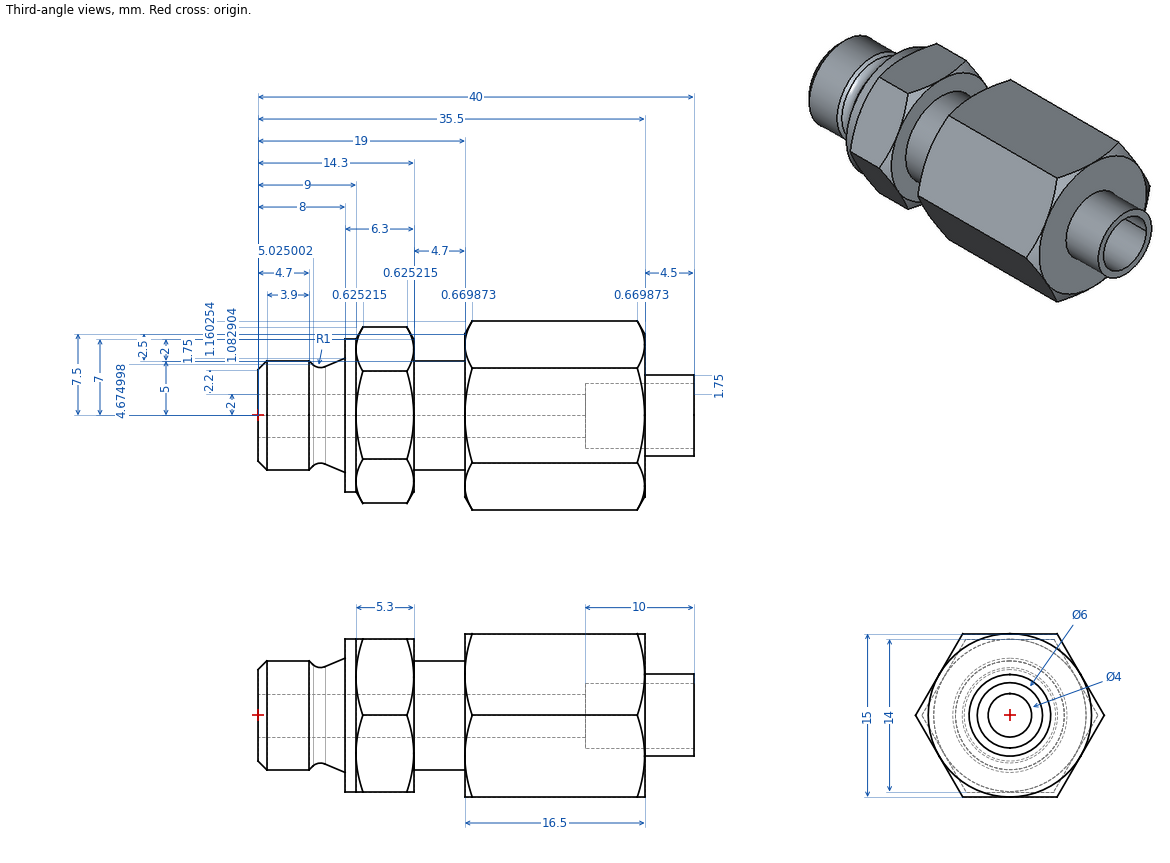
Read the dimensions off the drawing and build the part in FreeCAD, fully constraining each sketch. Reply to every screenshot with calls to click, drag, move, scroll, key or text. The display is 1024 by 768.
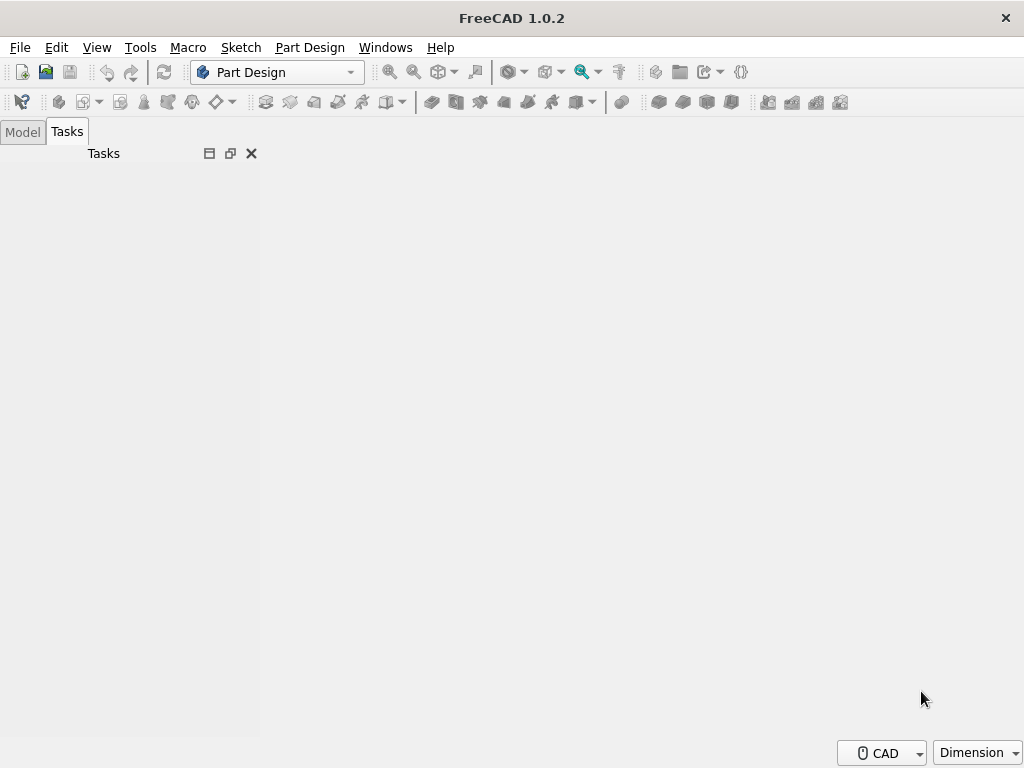
key(ctrl+n)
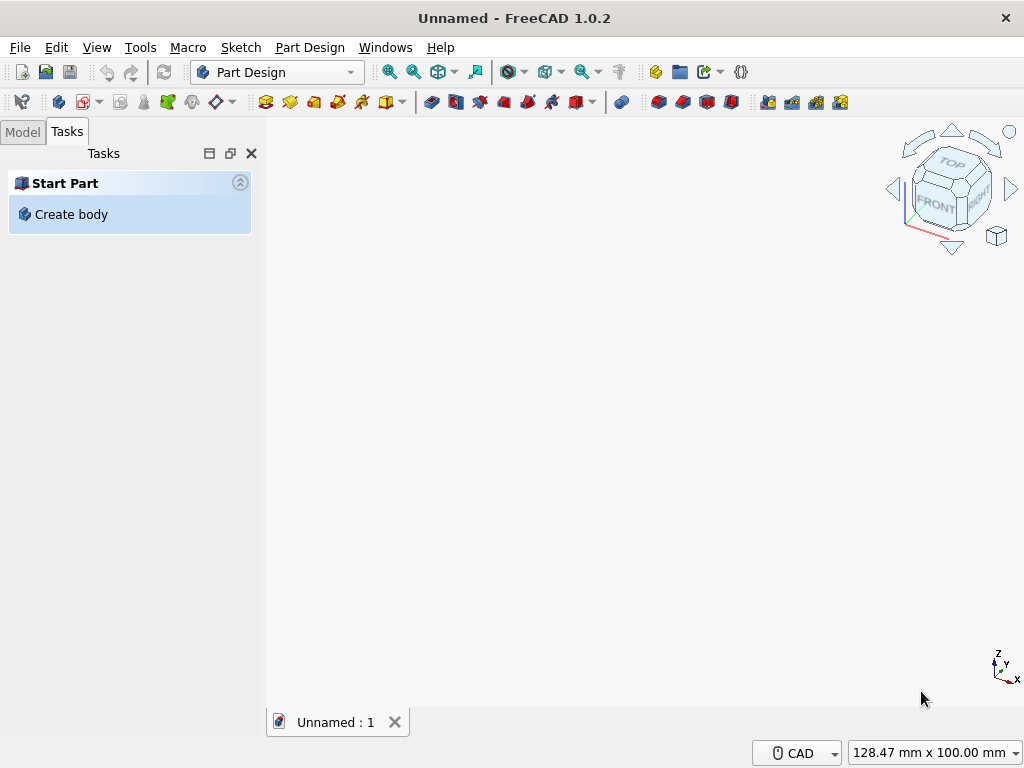
click(84, 102)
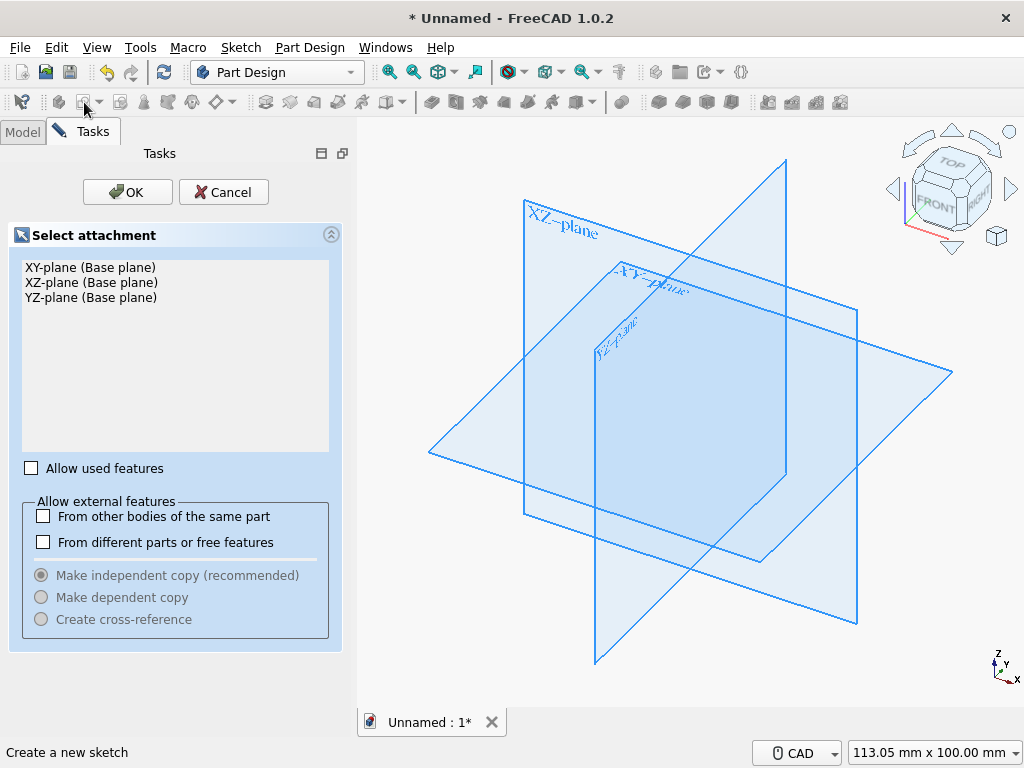
click(82, 268)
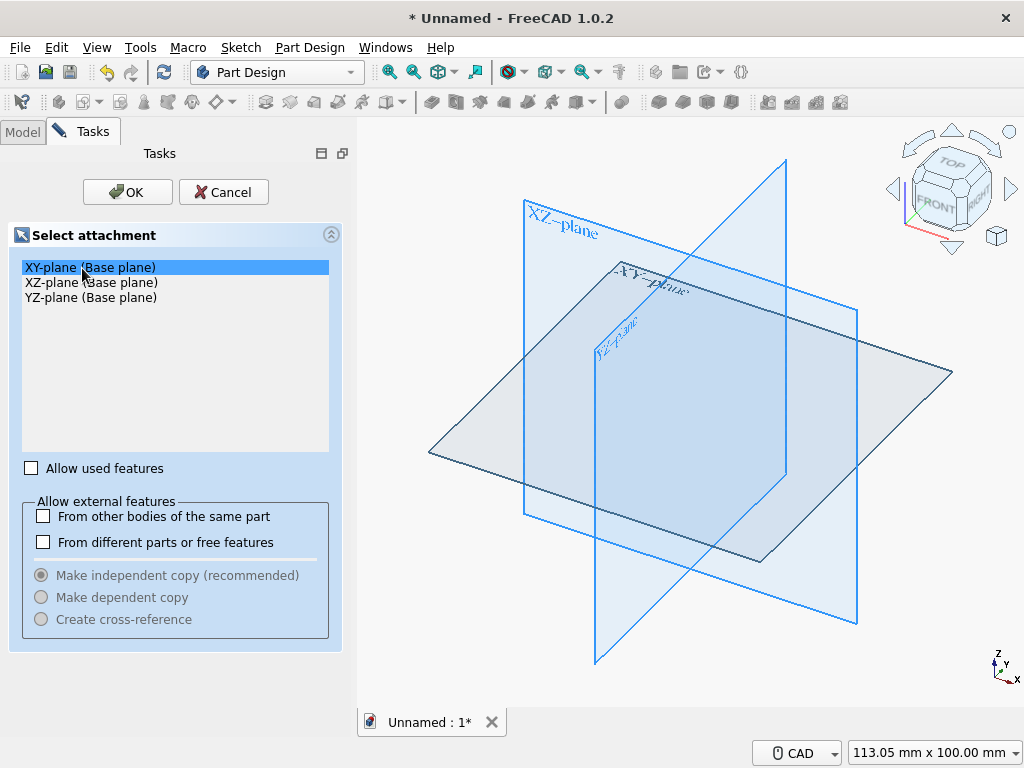
click(128, 192)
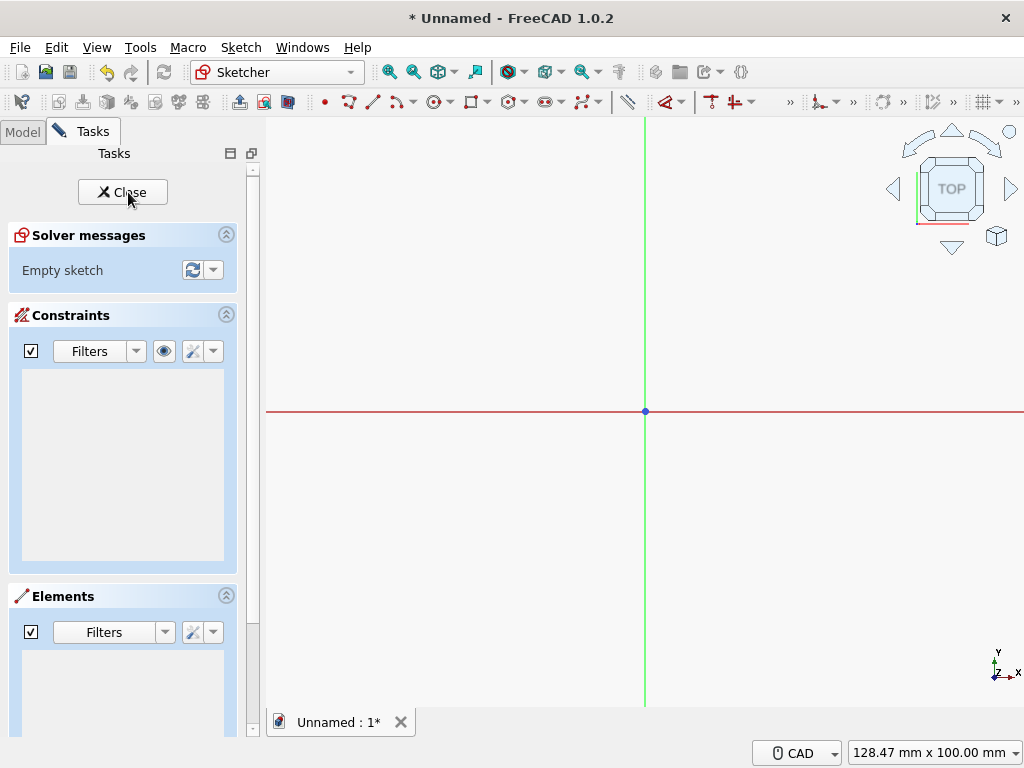
scroll(576, 412, down, 5)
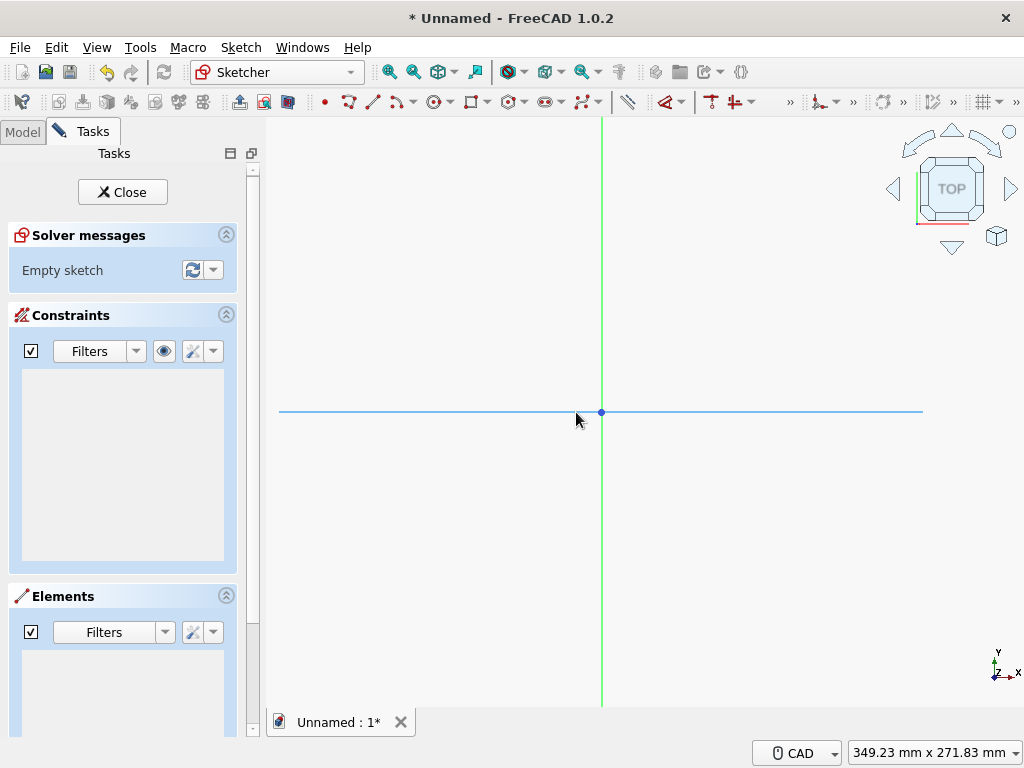
scroll(662, 402, up, 8)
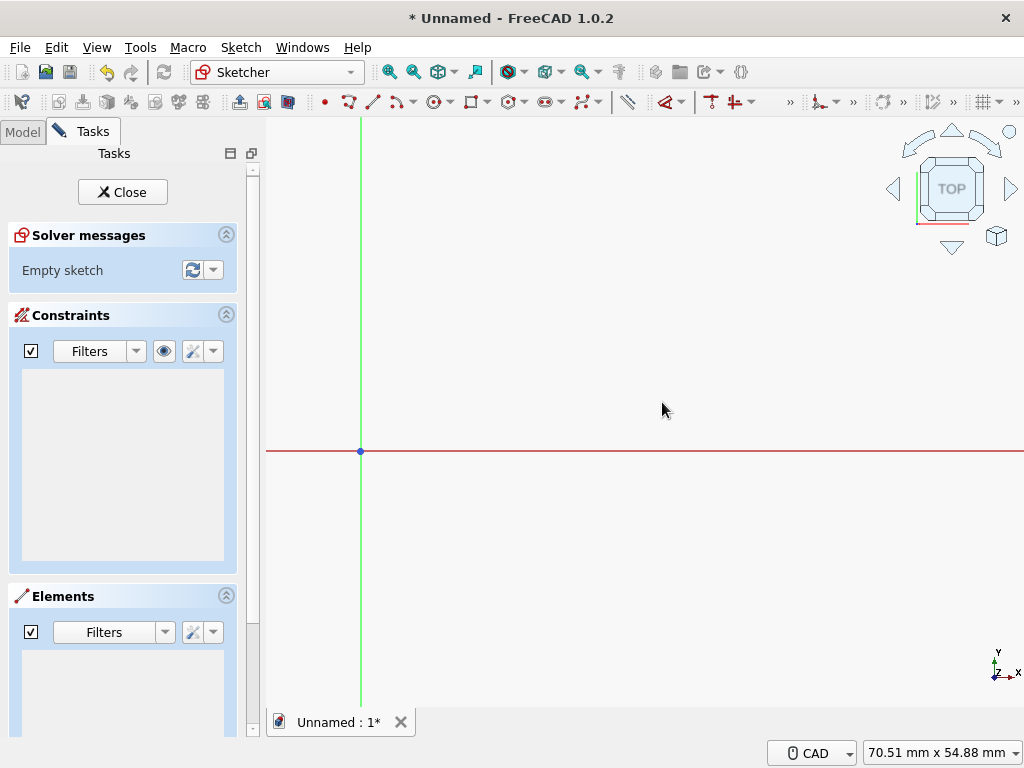
key(g)
key(m)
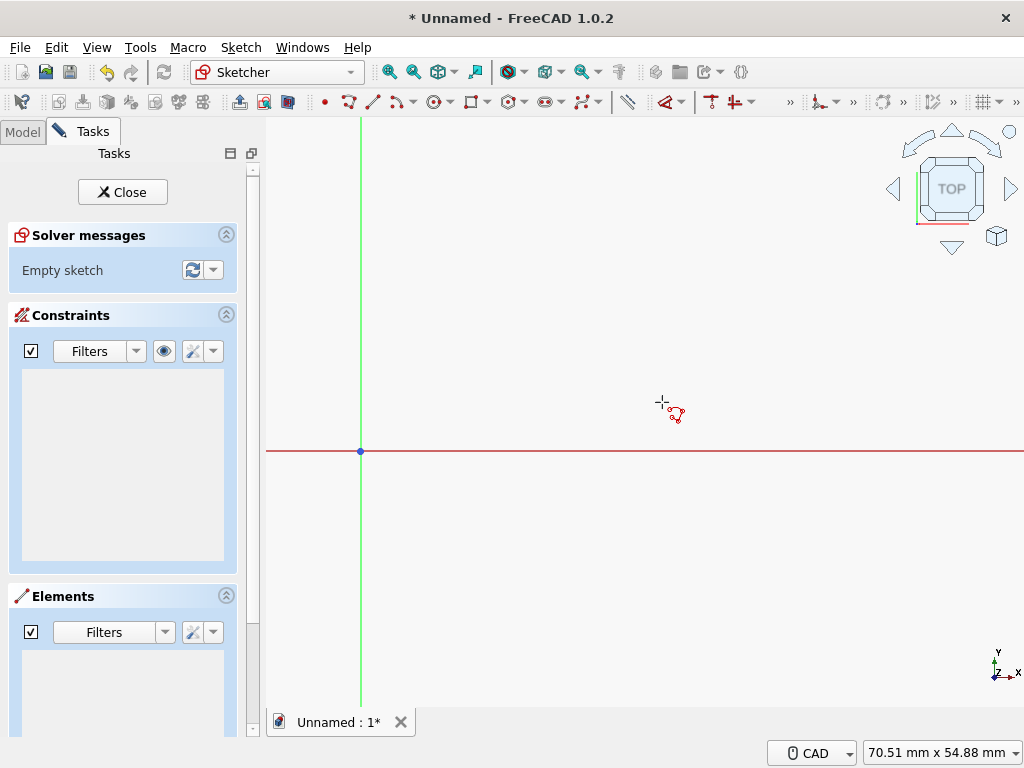
click(415, 401)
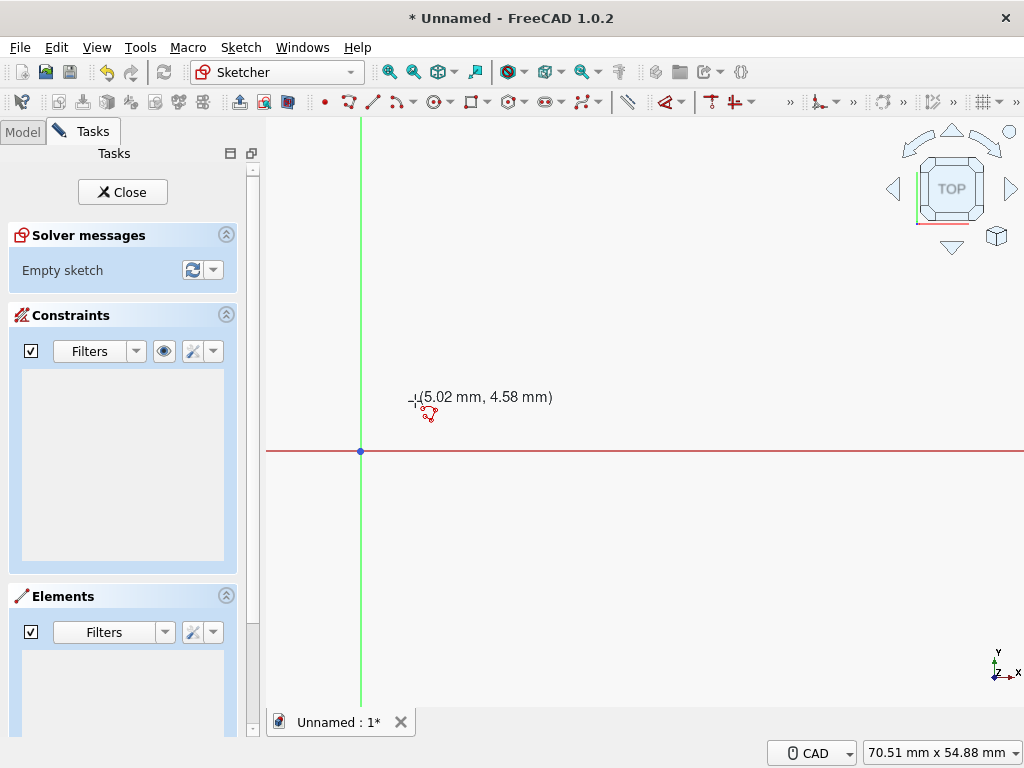
scroll(412, 397, up, 6)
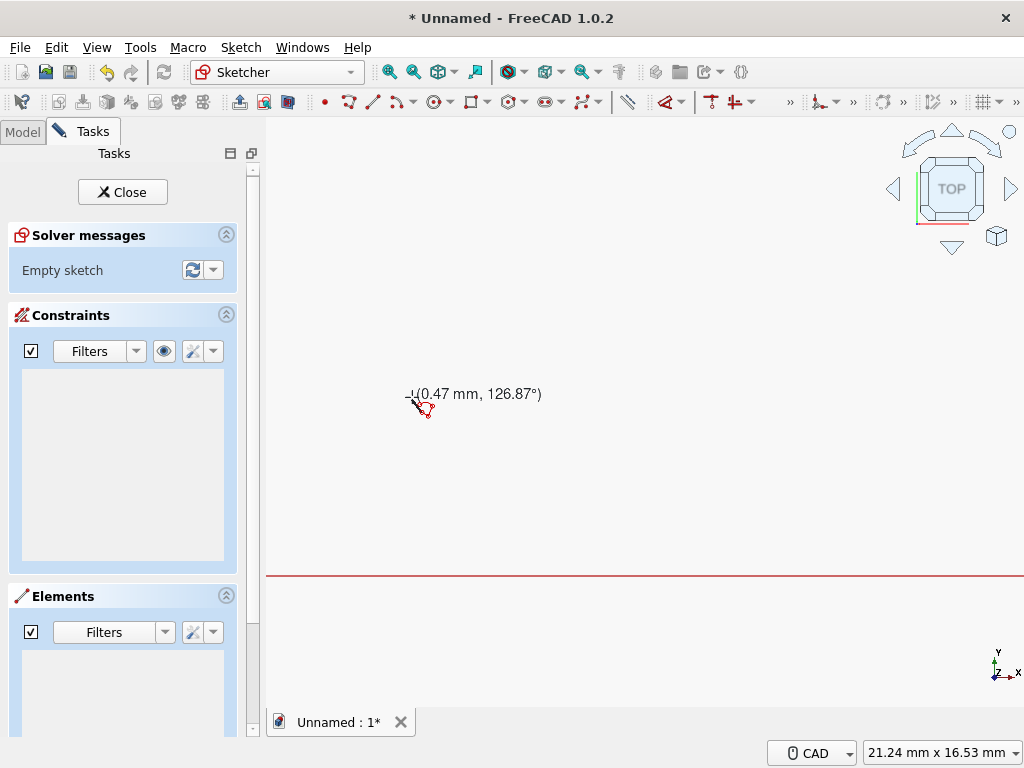
click(410, 397)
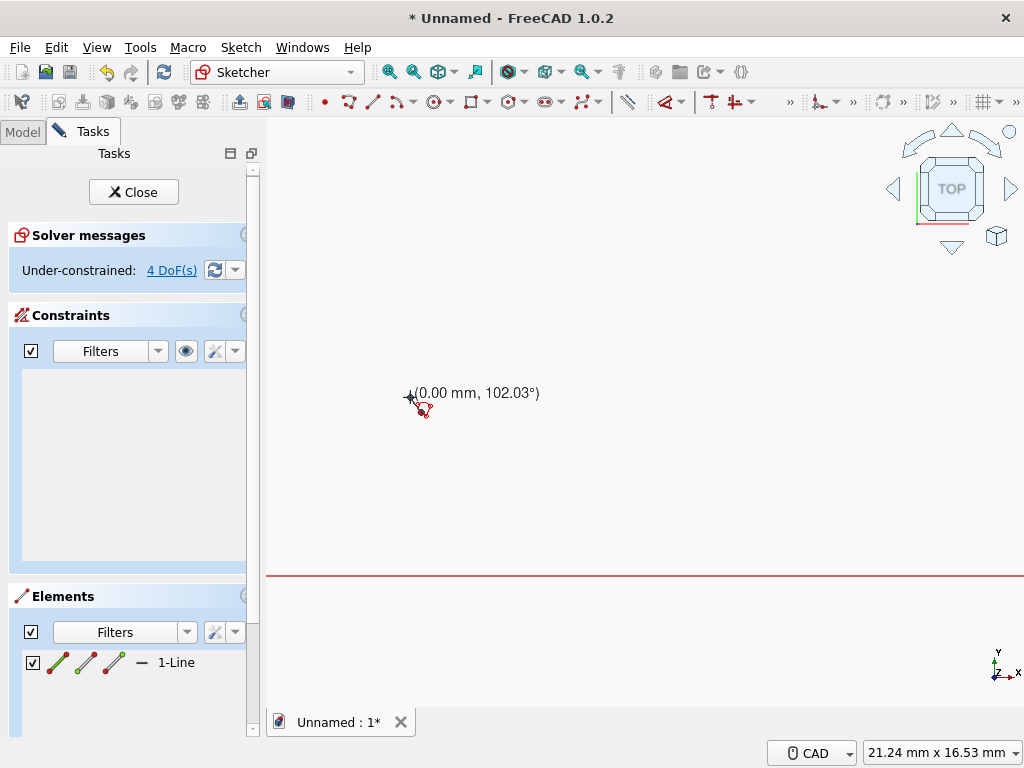
scroll(413, 399, down, 6)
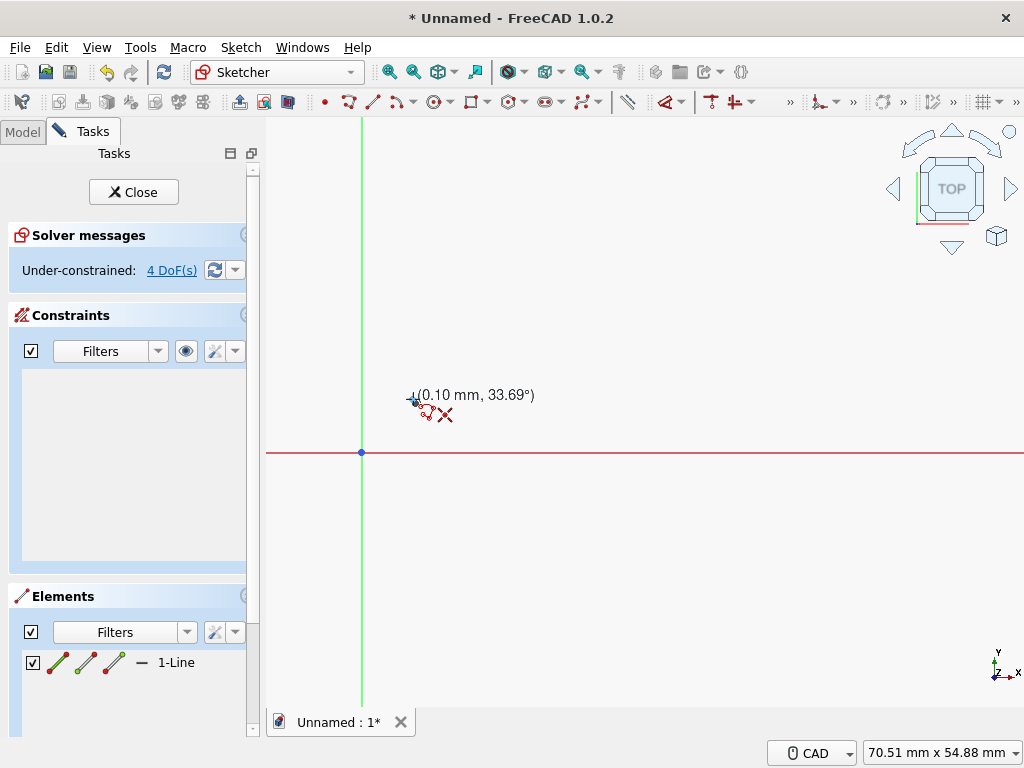
scroll(370, 399, up, 4)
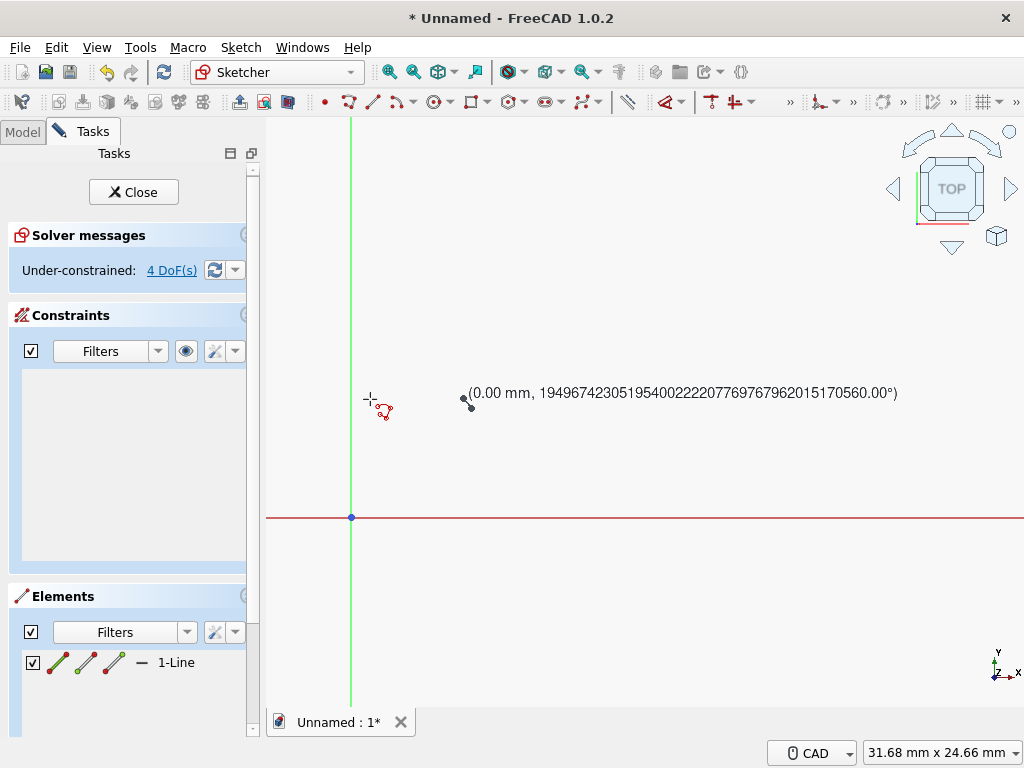
click(370, 398)
click(351, 417)
click(360, 470)